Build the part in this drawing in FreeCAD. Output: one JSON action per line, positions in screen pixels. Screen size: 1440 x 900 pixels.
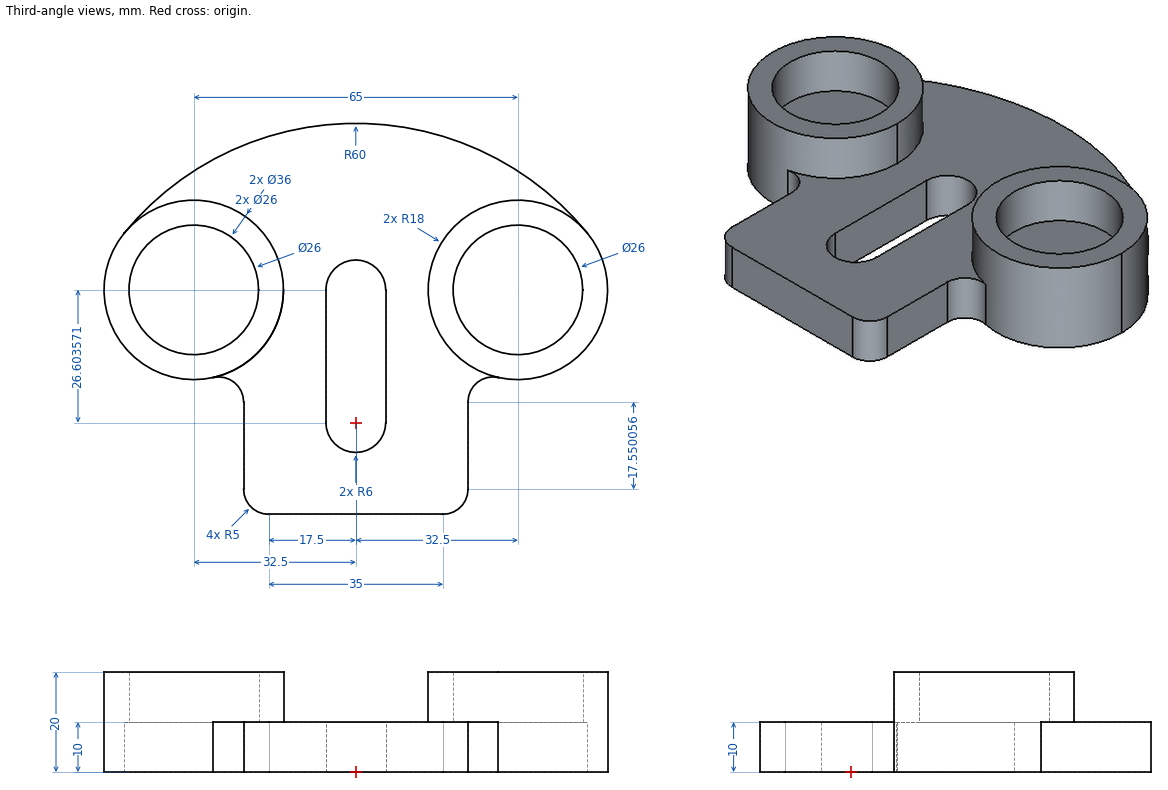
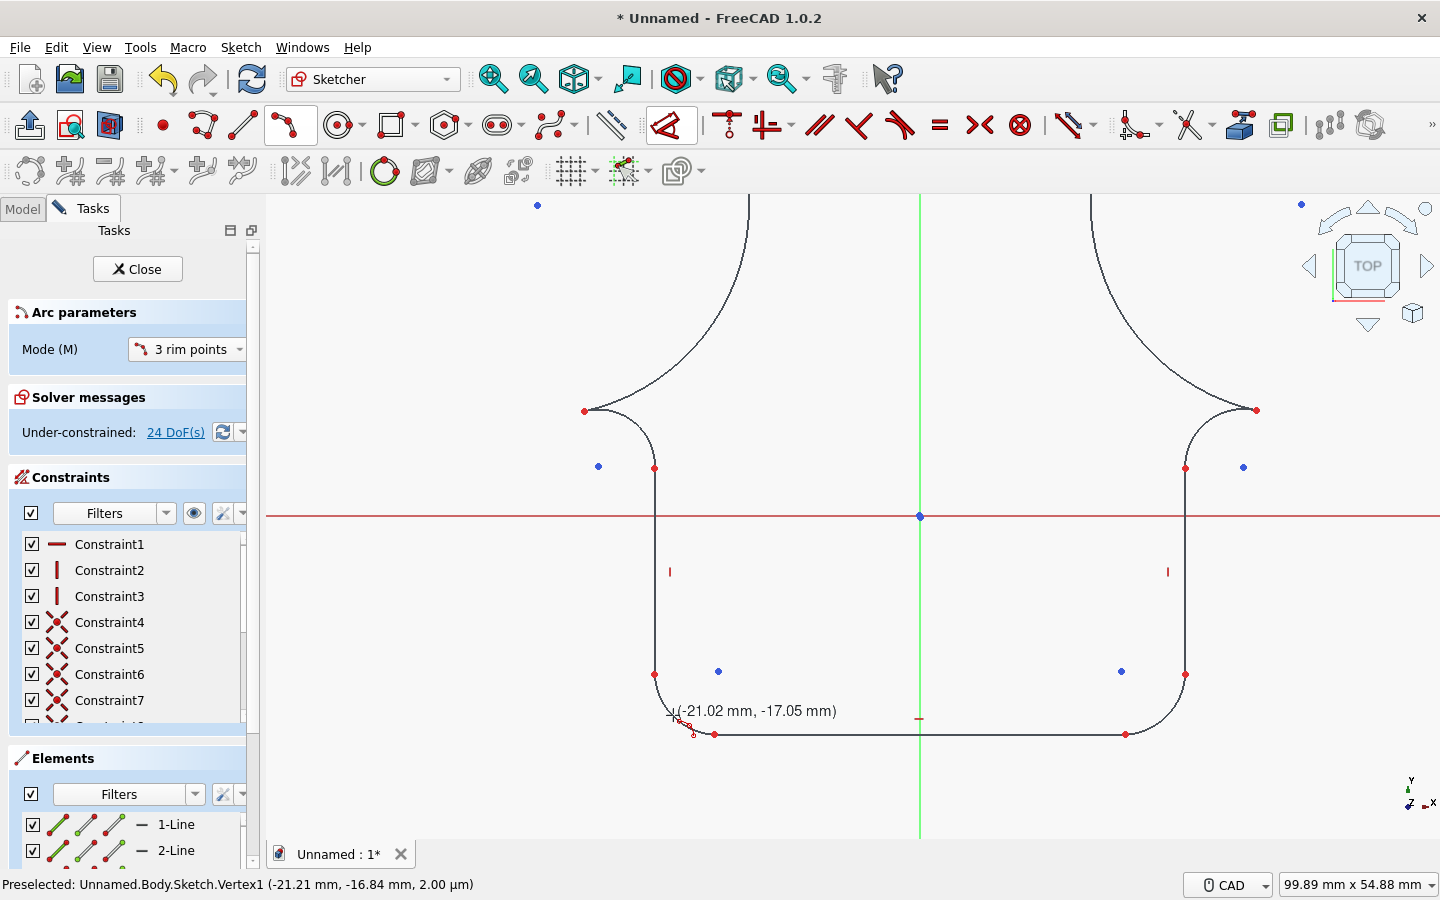
{"action": "left_click", "coordinate": [498, 126]}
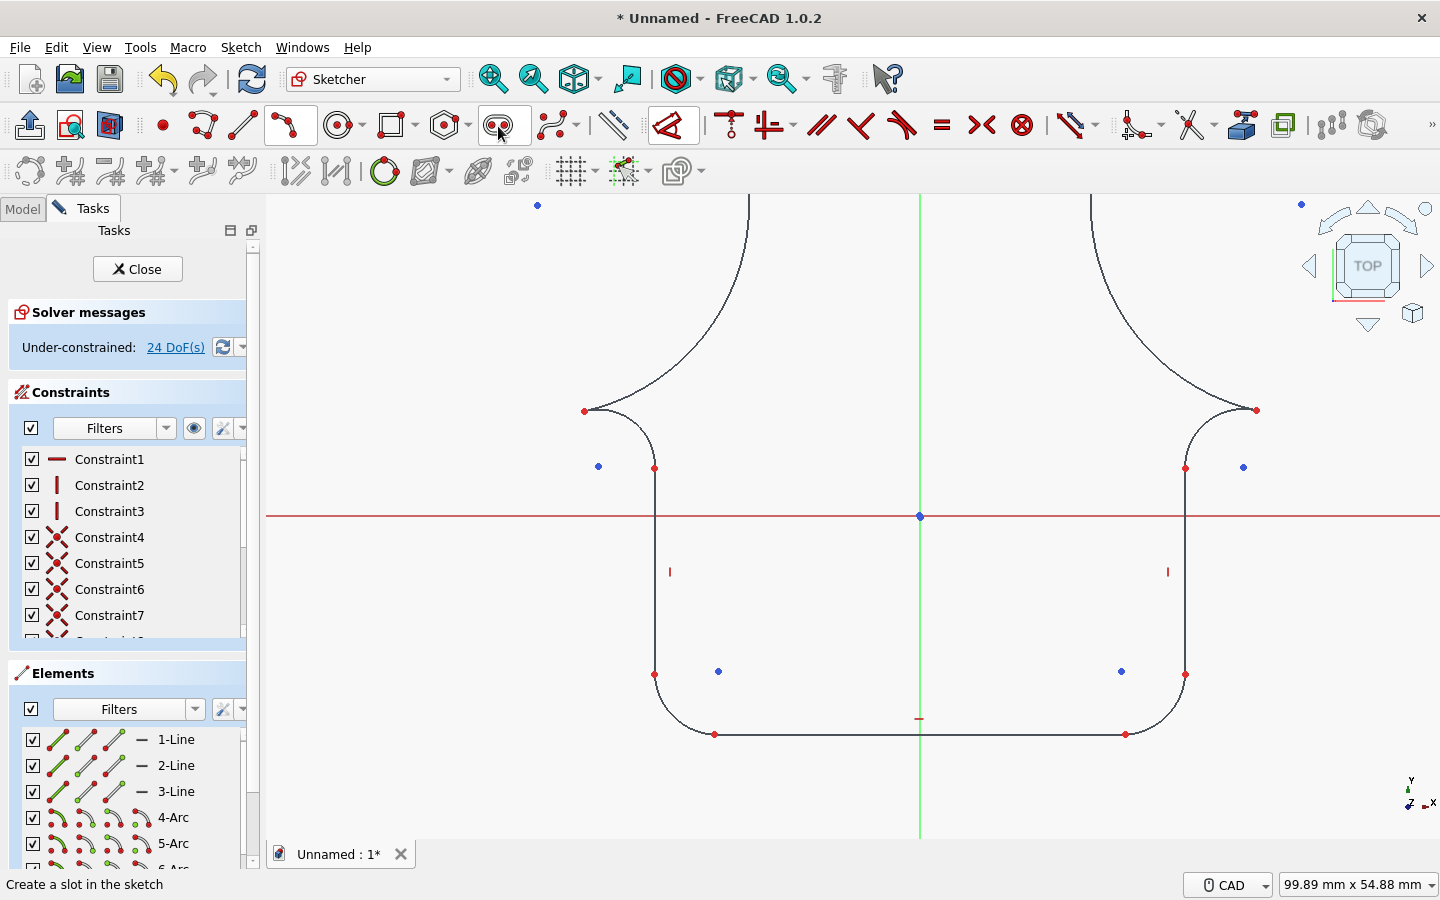
{"action": "left_click", "coordinate": [920, 516]}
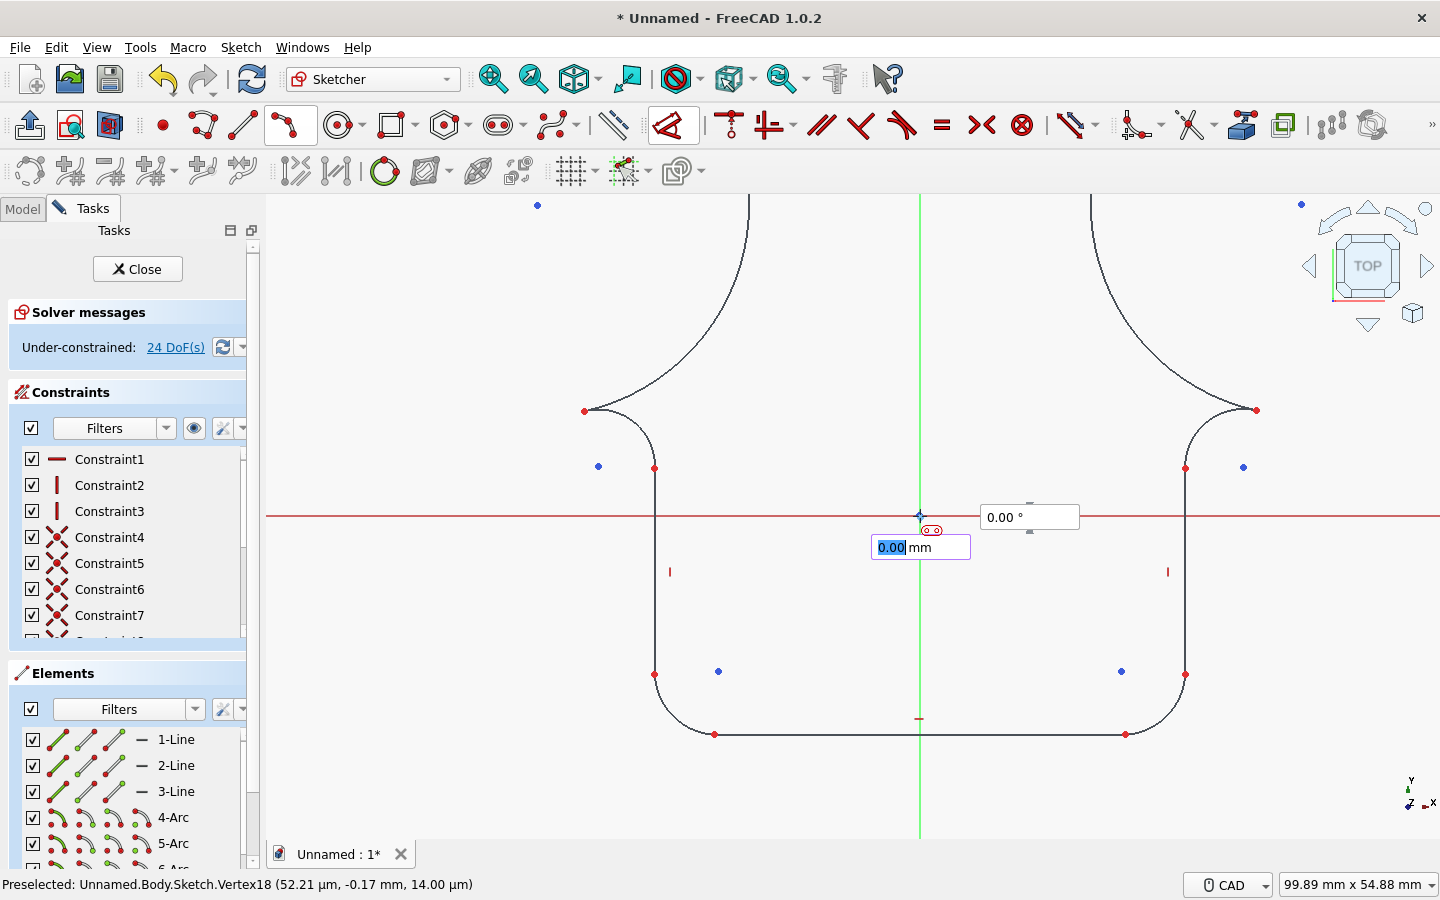
{"action": "scroll", "coordinate": [674, 717], "scroll_direction": "down", "scroll_amount": 4}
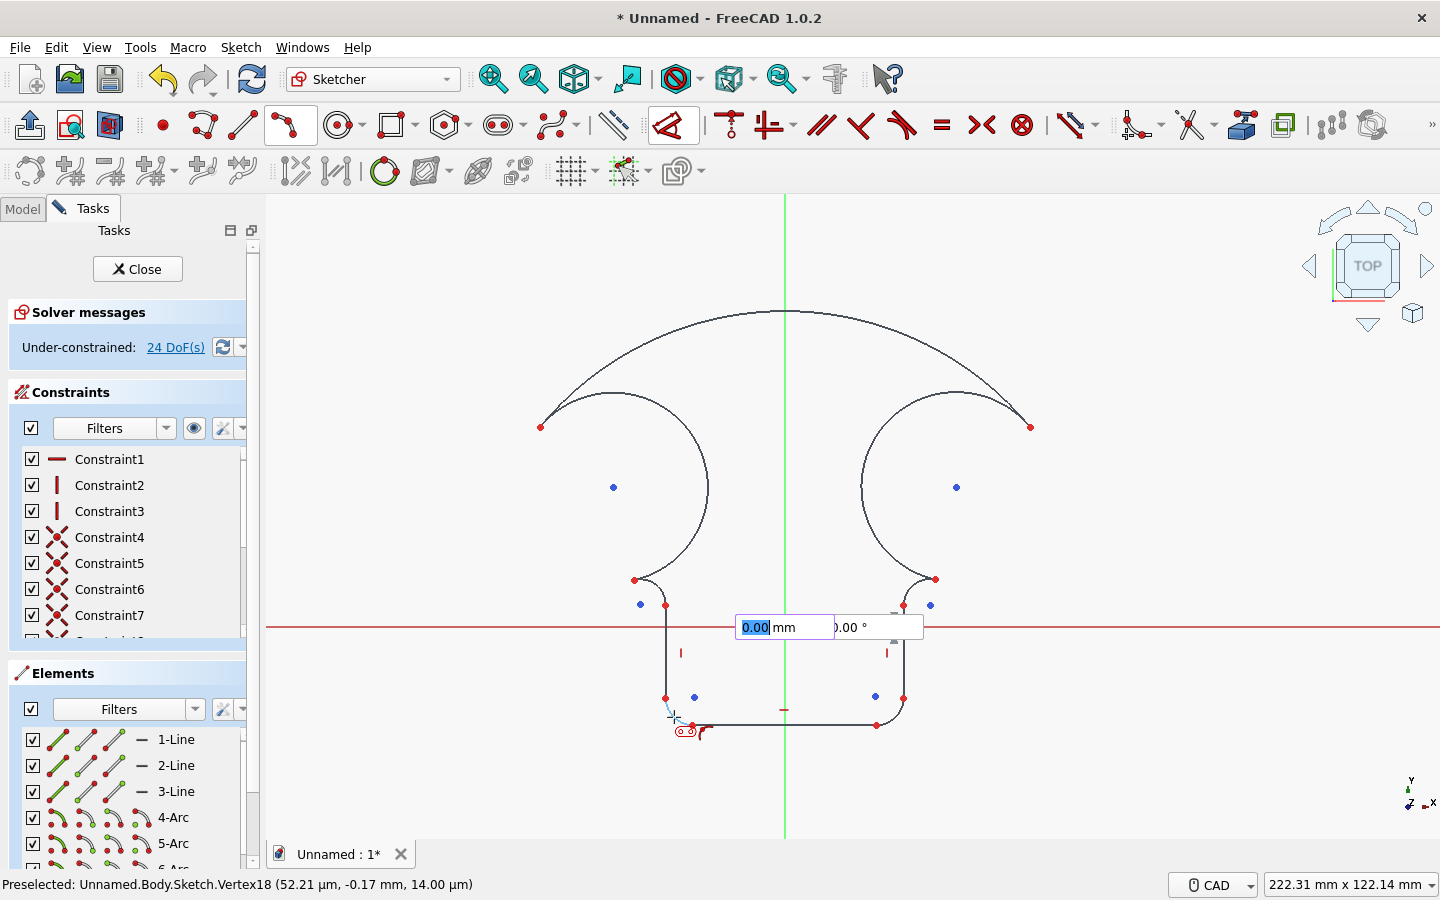
{"action": "left_click", "coordinate": [794, 486]}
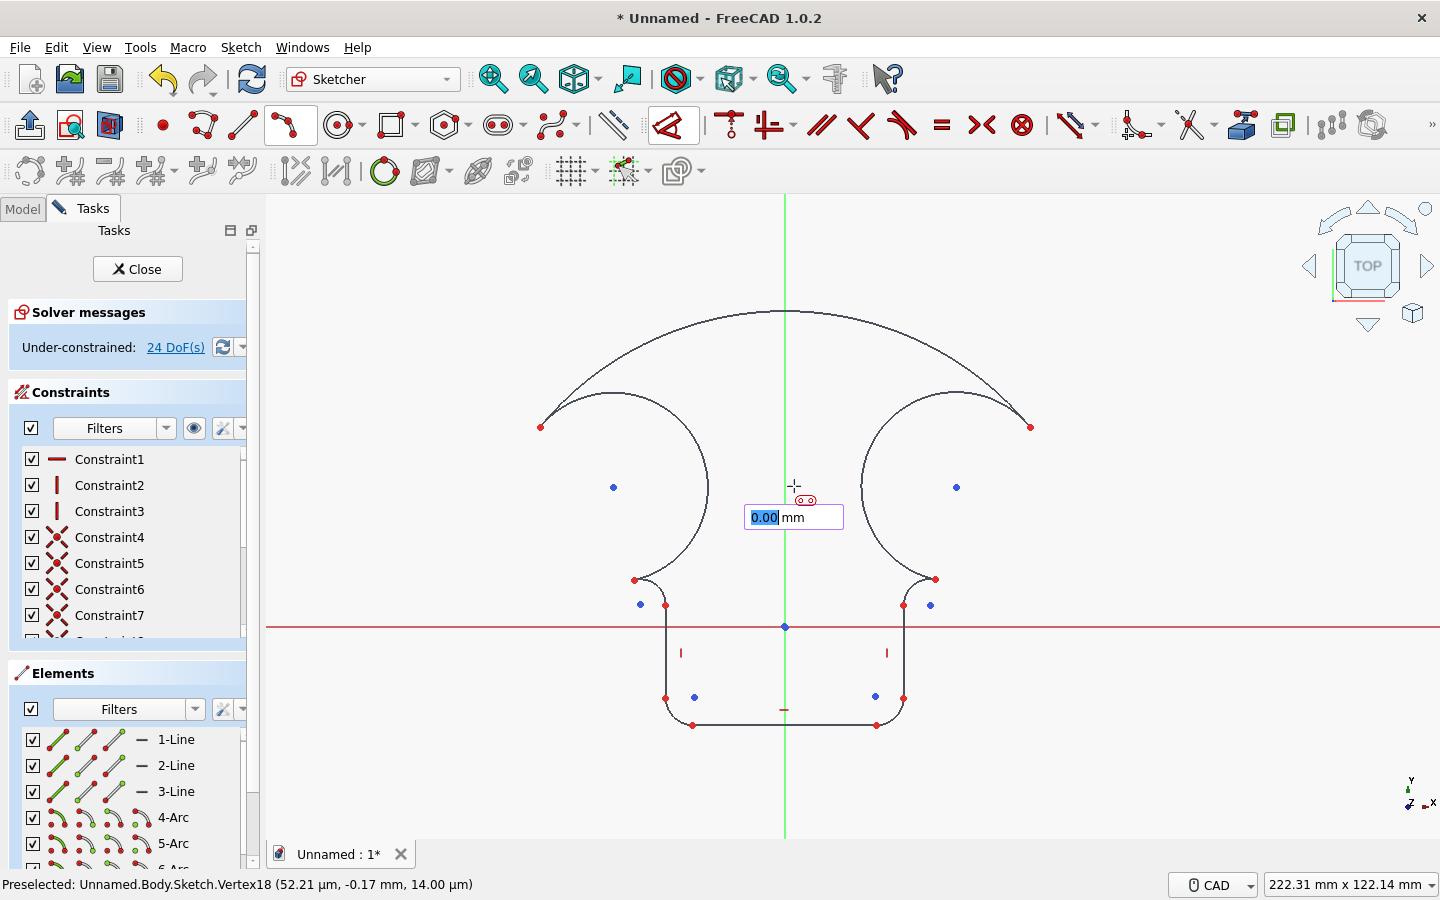
{"action": "left_click", "coordinate": [753, 557]}
{"action": "key", "text": "Escape"}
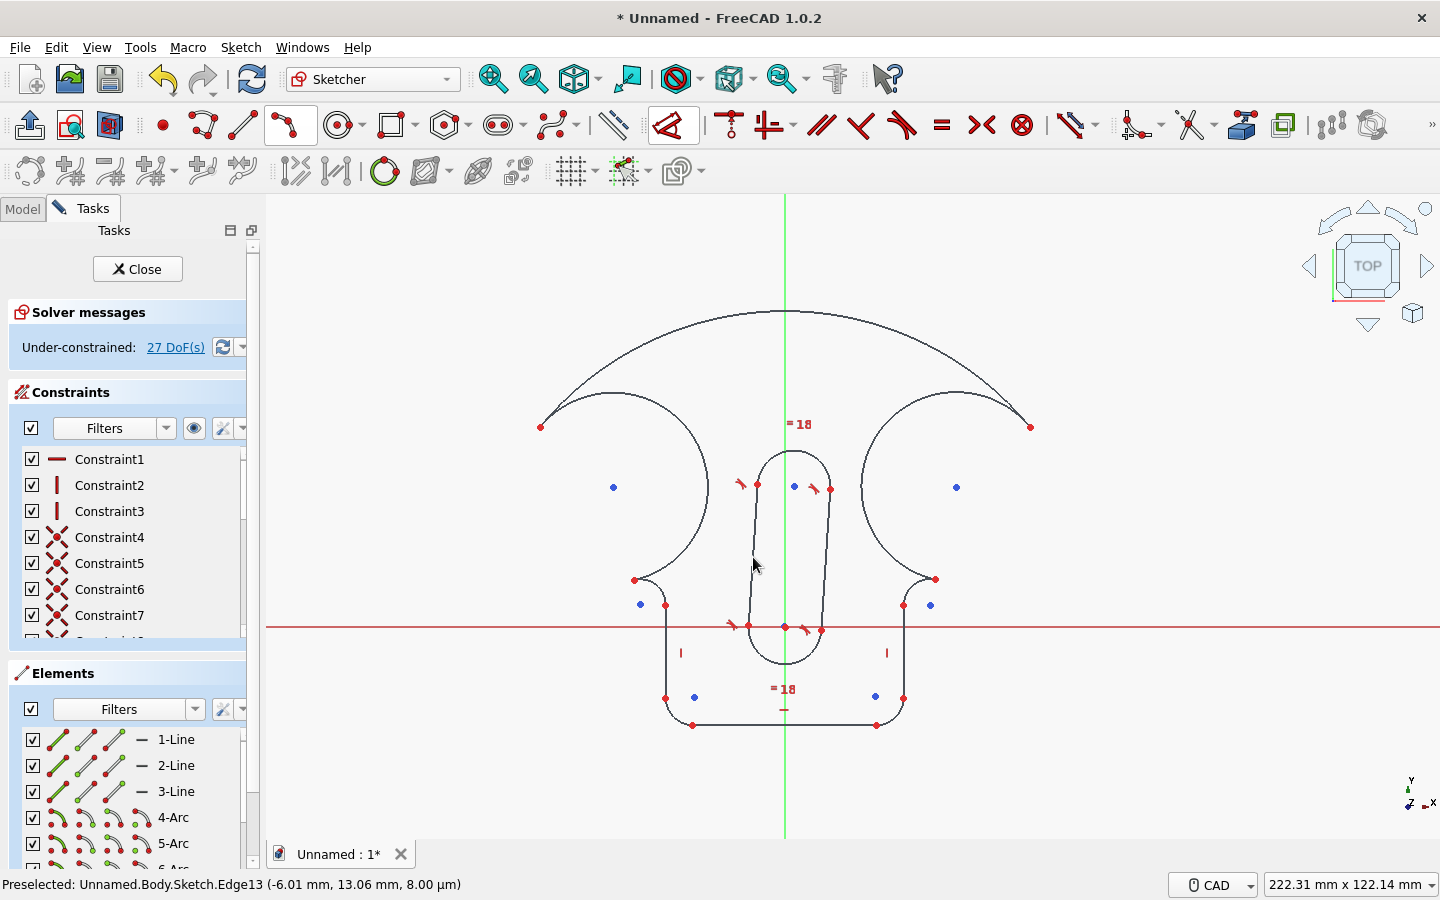
{"action": "left_click", "coordinate": [748, 725]}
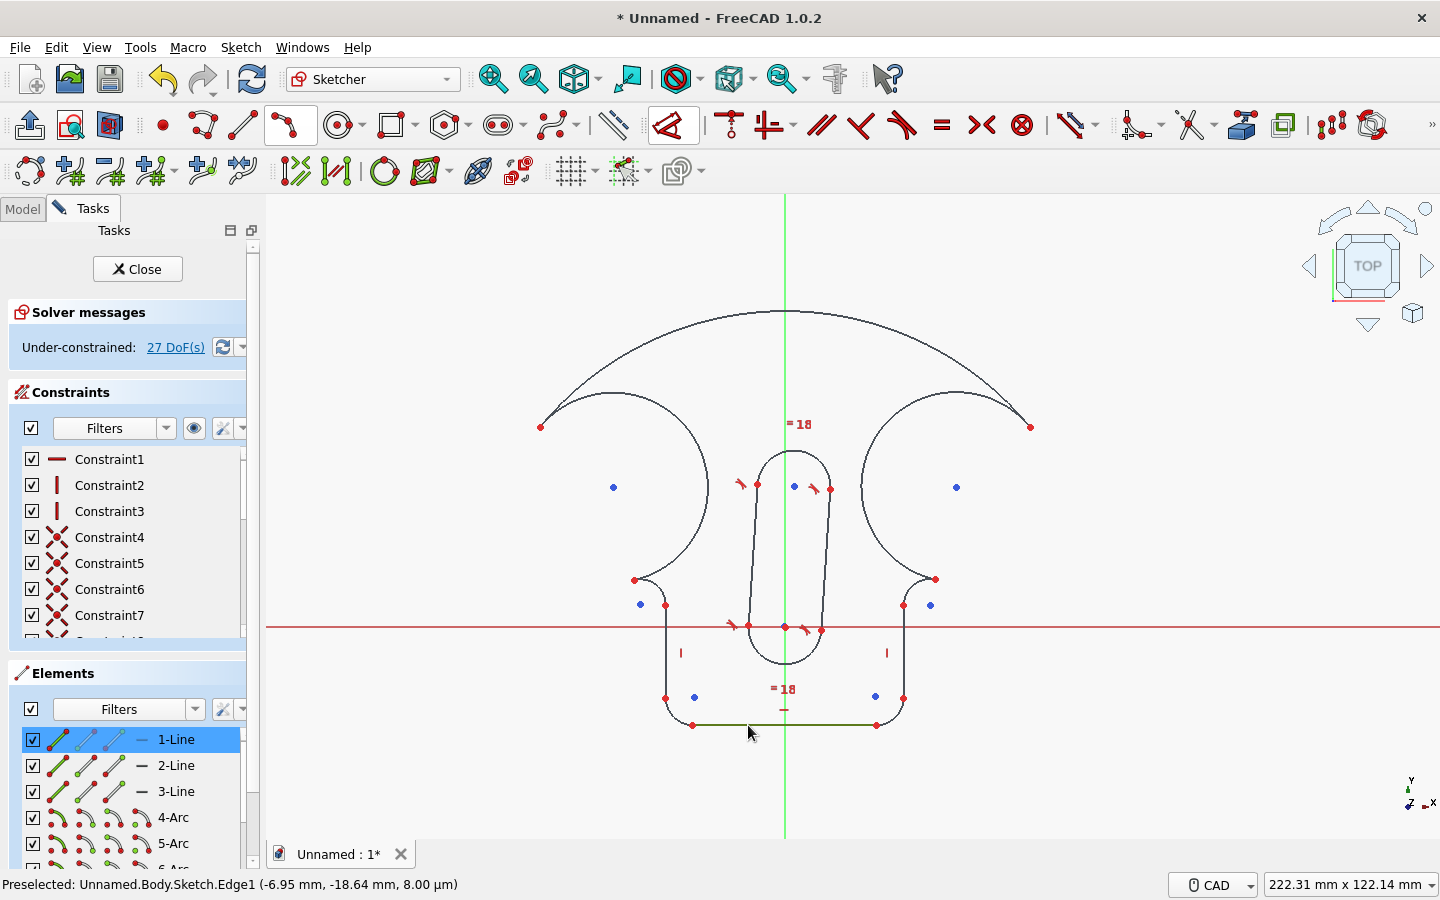
{"action": "left_click", "coordinate": [889, 722]}